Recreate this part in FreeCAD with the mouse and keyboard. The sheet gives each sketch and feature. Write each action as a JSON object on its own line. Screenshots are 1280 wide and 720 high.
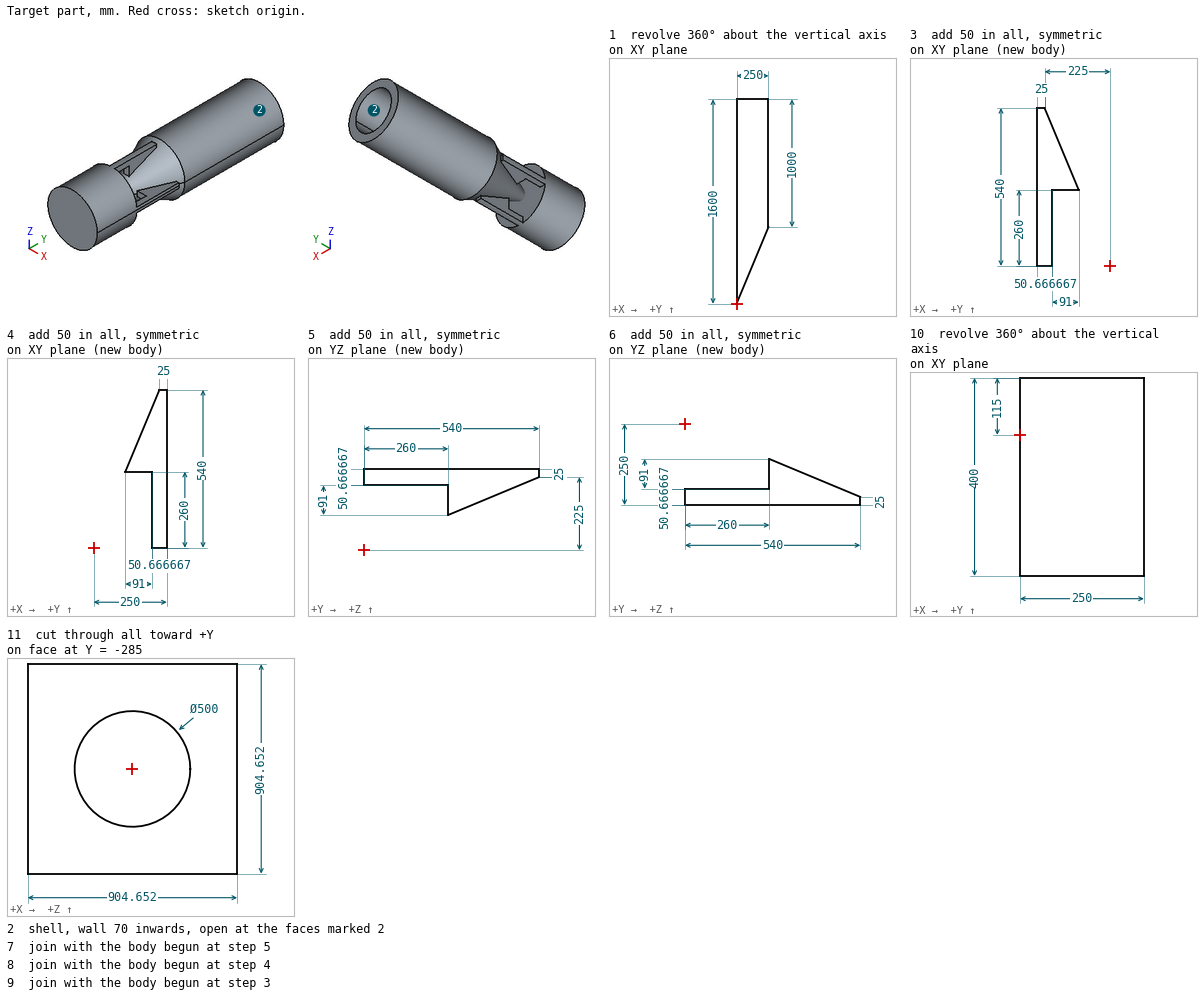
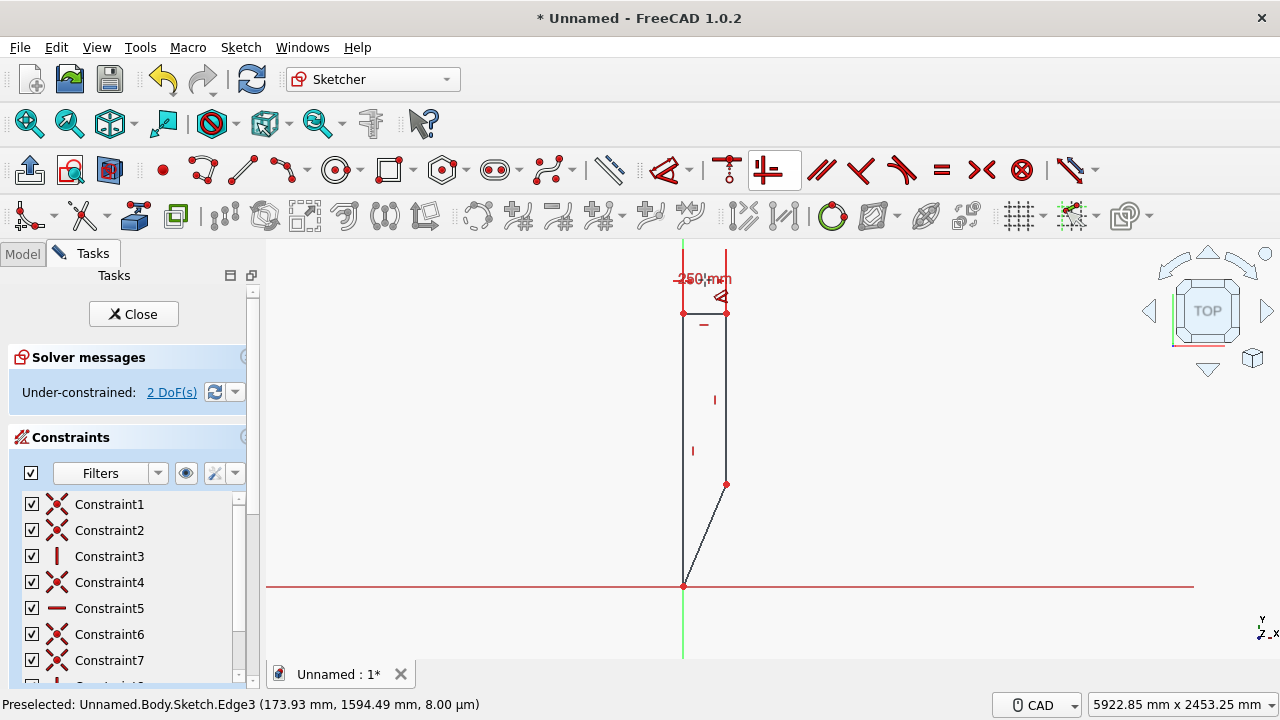
{"action": "left_click", "coordinate": [726, 434]}
{"action": "left_click", "coordinate": [760, 399]}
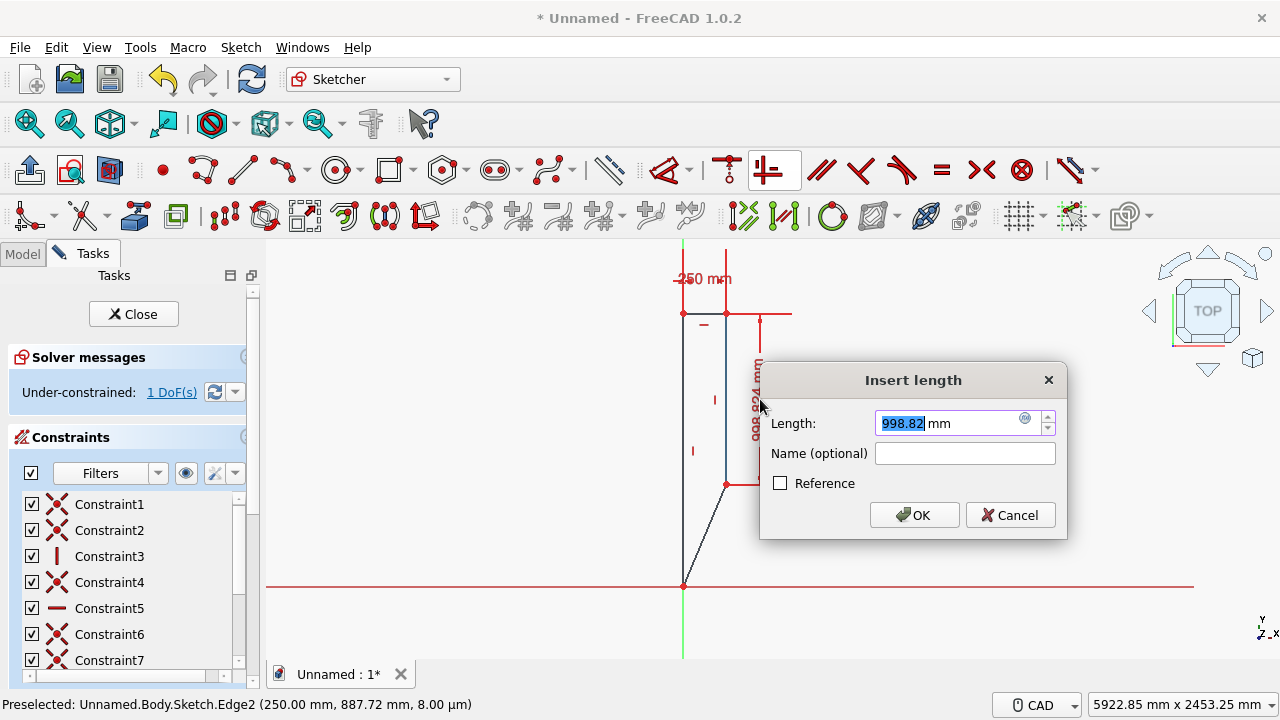
{"action": "type", "text": "1000"}
{"action": "key", "text": "Return"}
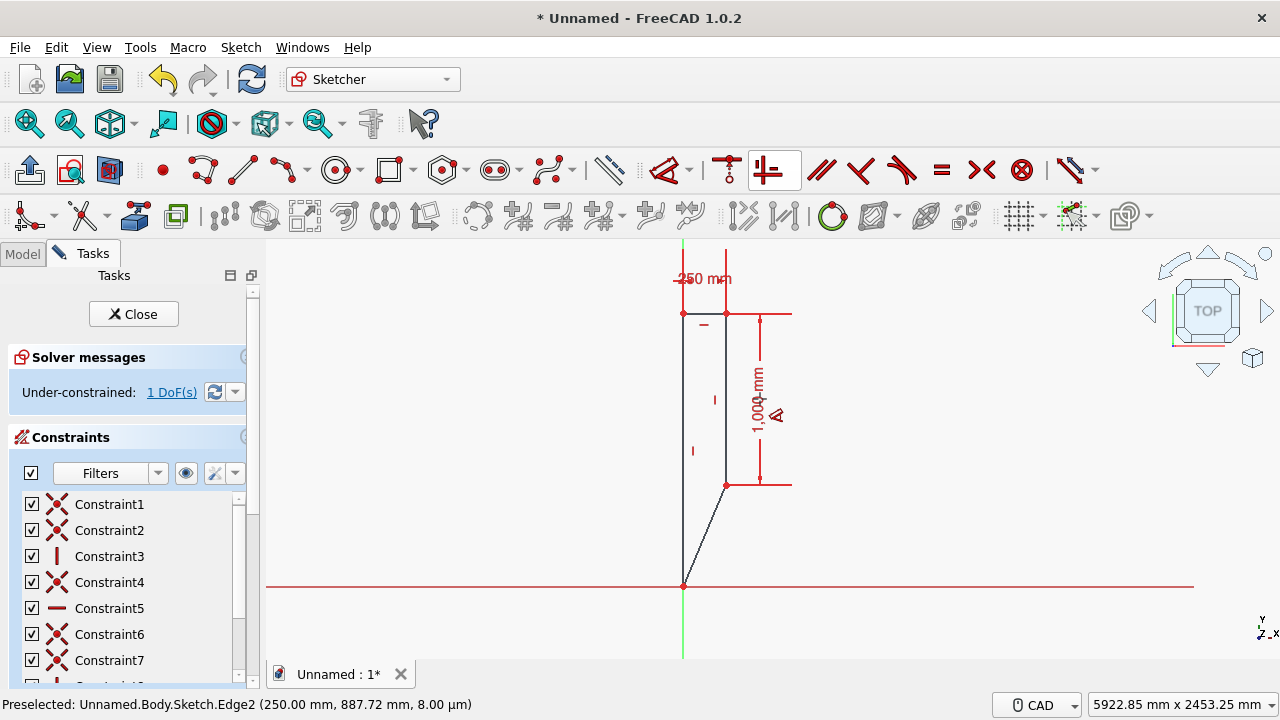
{"action": "left_click", "coordinate": [683, 396]}
{"action": "left_click", "coordinate": [649, 450]}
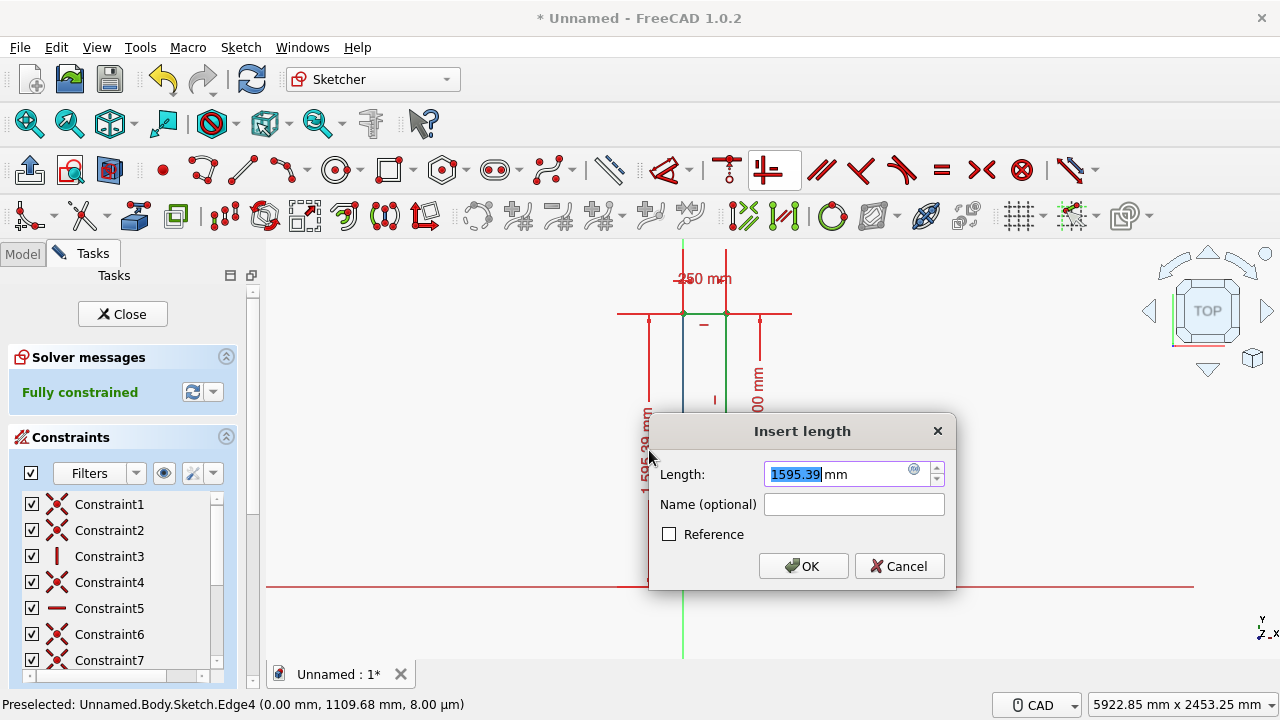
{"action": "type", "text": "1600"}
{"action": "key", "text": "Return"}
{"action": "key", "text": "Escape"}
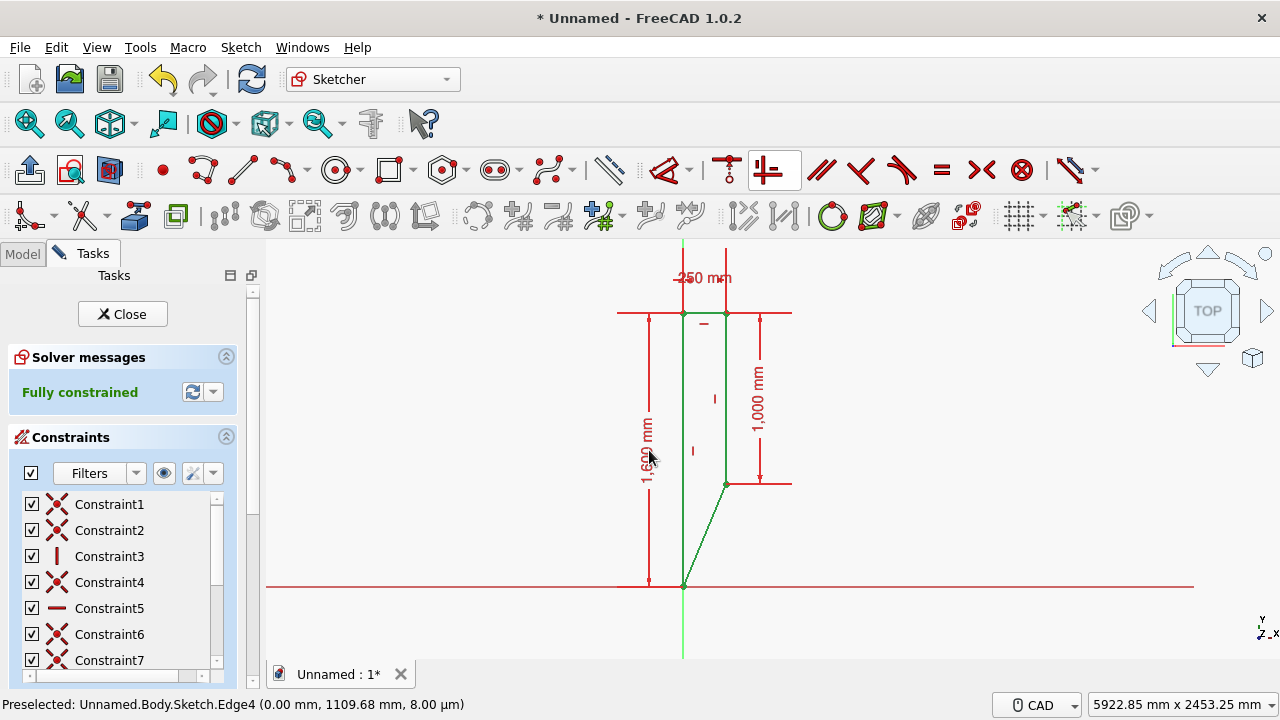
{"action": "left_click", "coordinate": [123, 314]}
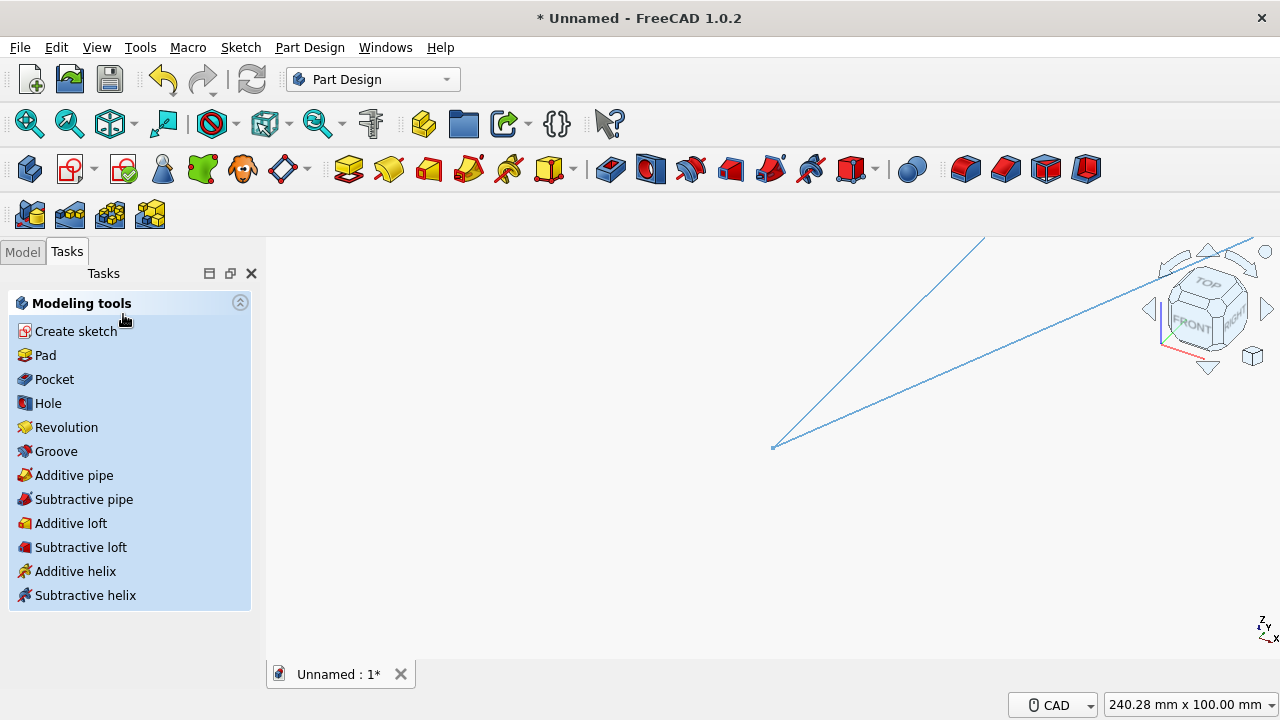
{"action": "left_click", "coordinate": [390, 170]}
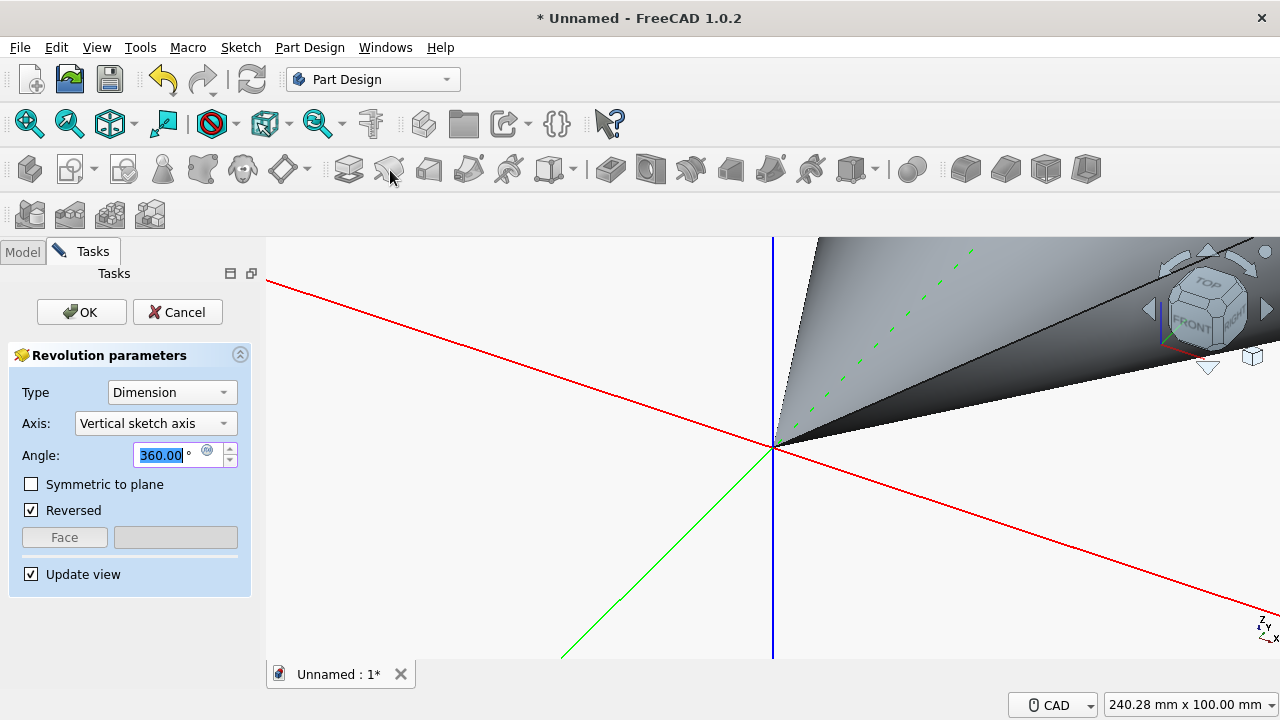
{"action": "left_click", "coordinate": [82, 312]}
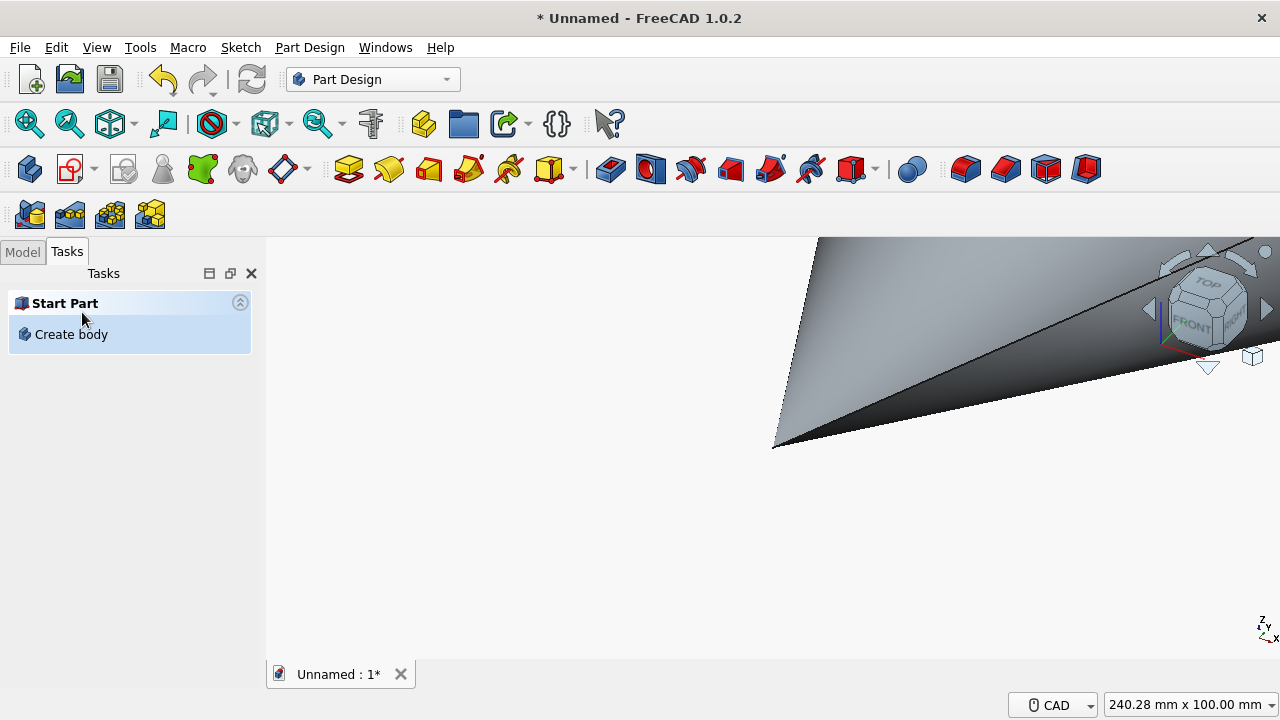
{"action": "left_click", "coordinate": [30, 124]}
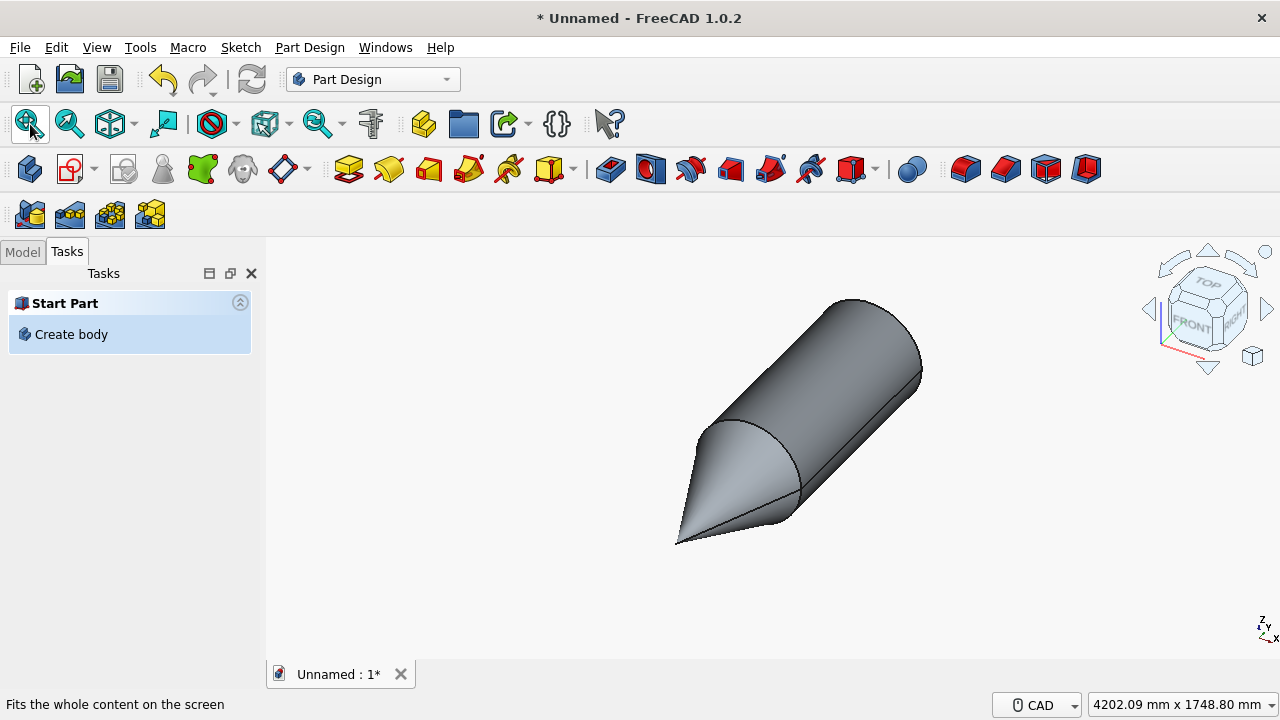
{"action": "key", "text": "0"}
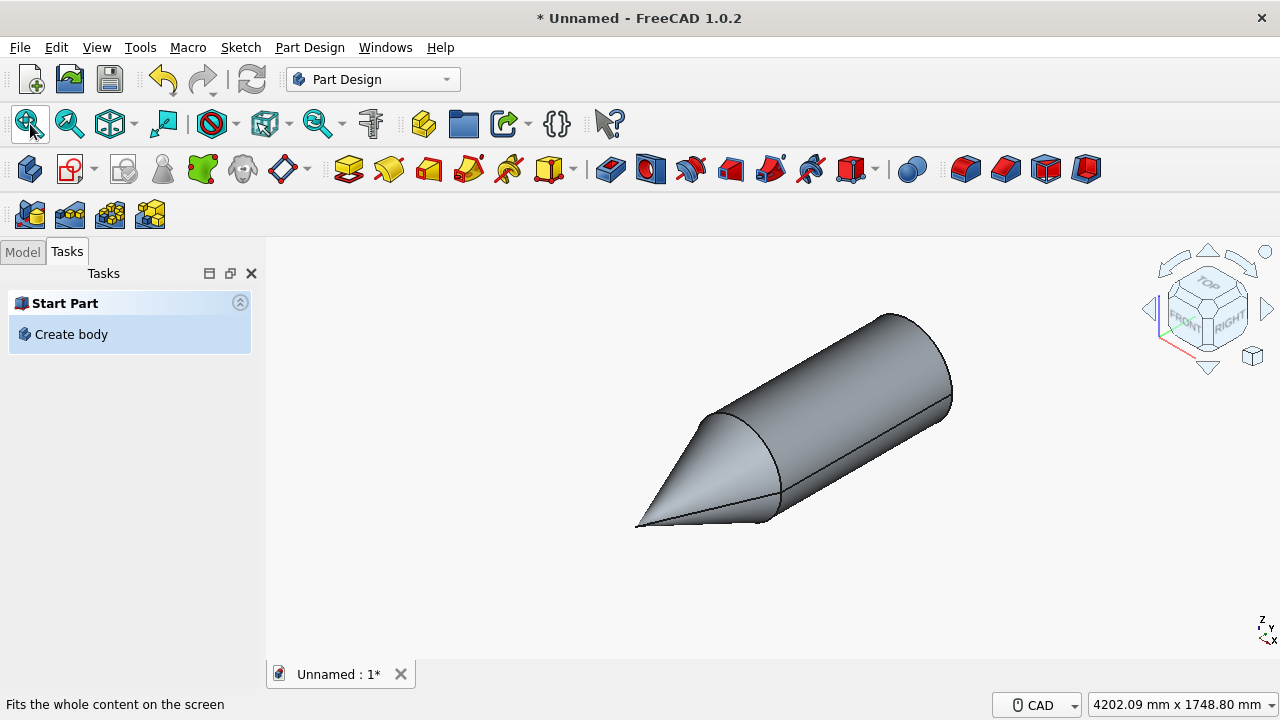
{"action": "key", "text": "2"}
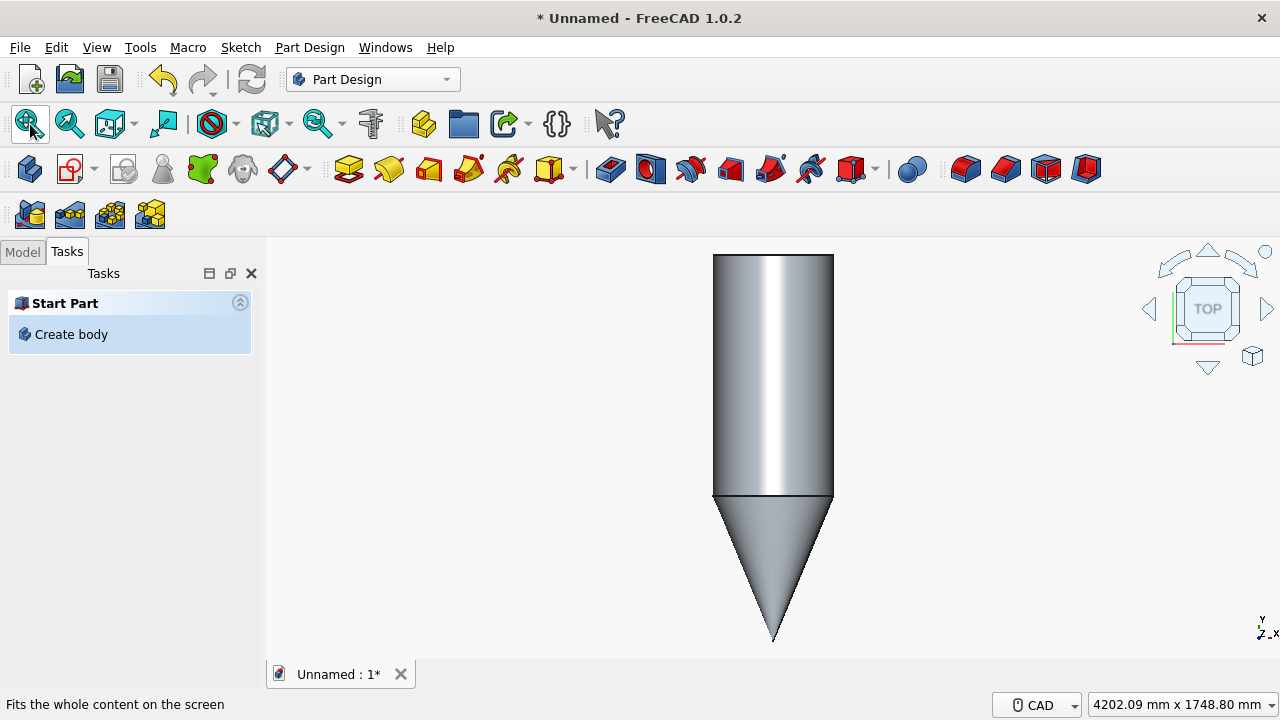
{"action": "key", "text": "1"}